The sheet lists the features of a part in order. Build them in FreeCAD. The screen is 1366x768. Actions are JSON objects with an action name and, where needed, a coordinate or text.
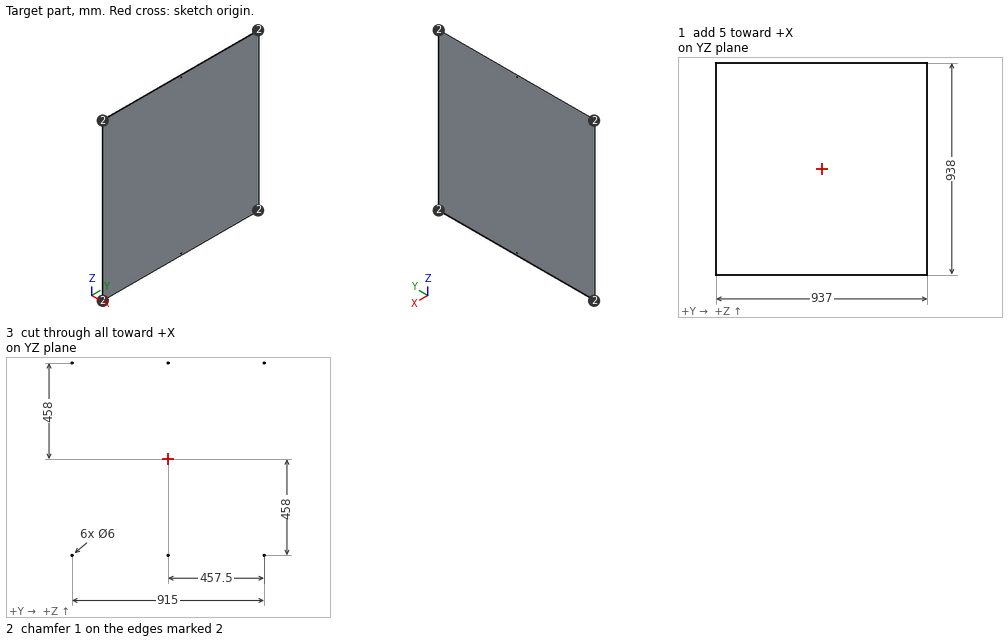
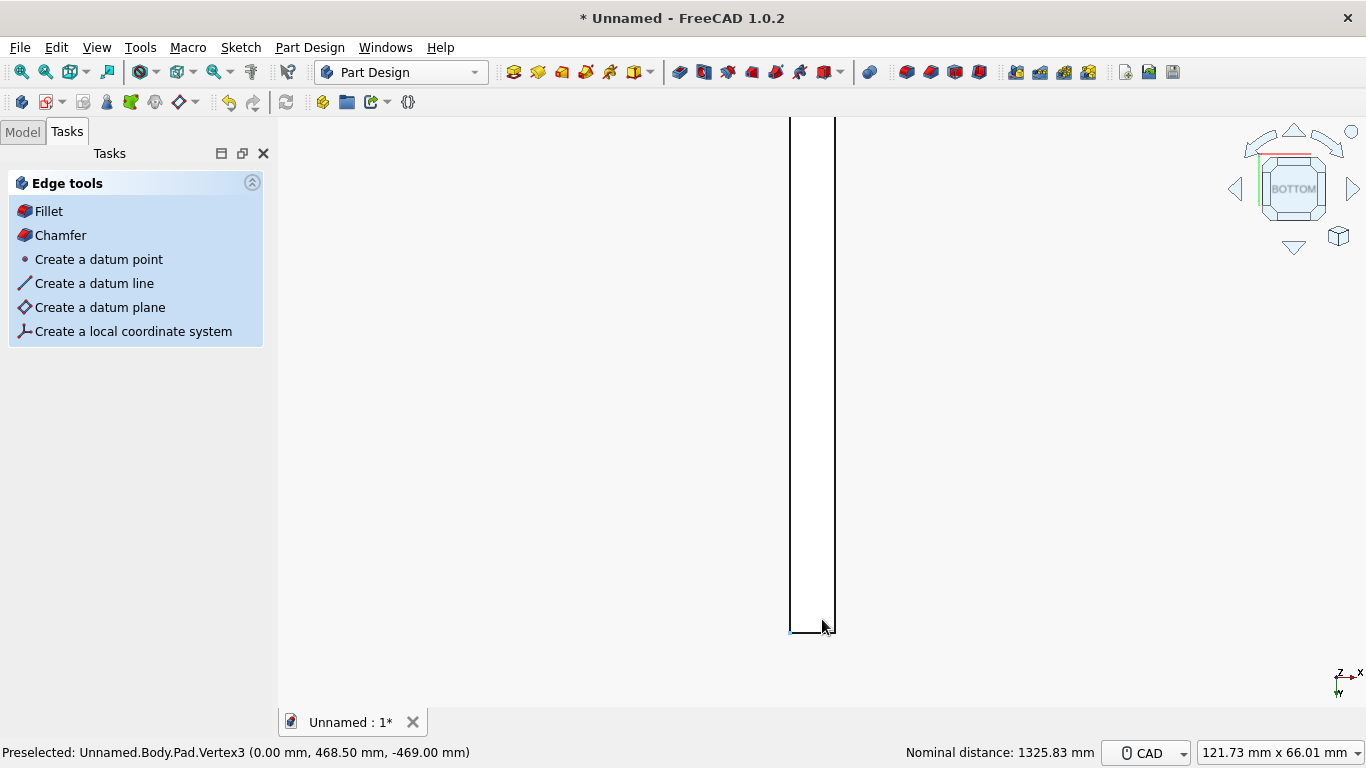
{"action": "left_click", "coordinate": [812, 632], "text": "ctrl"}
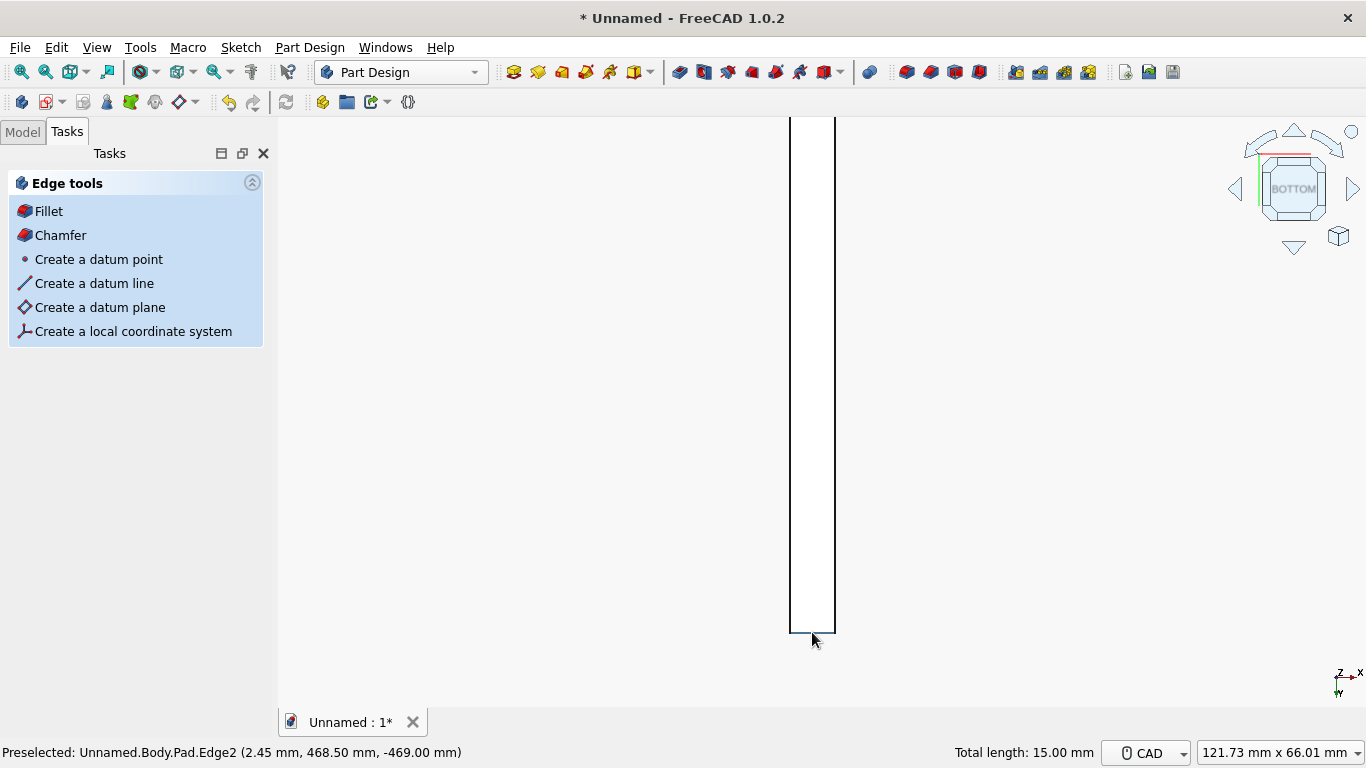
{"action": "left_click", "coordinate": [22, 72]}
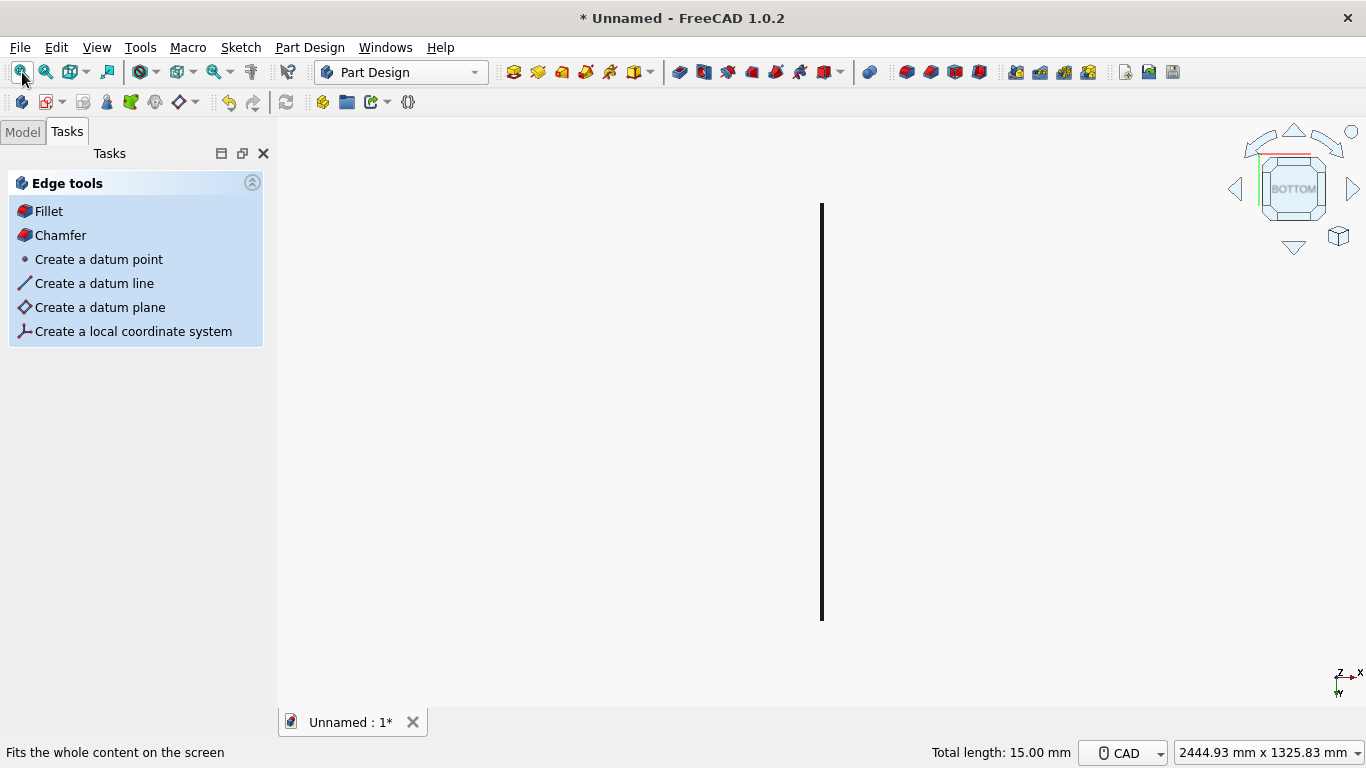
{"action": "key", "text": "4"}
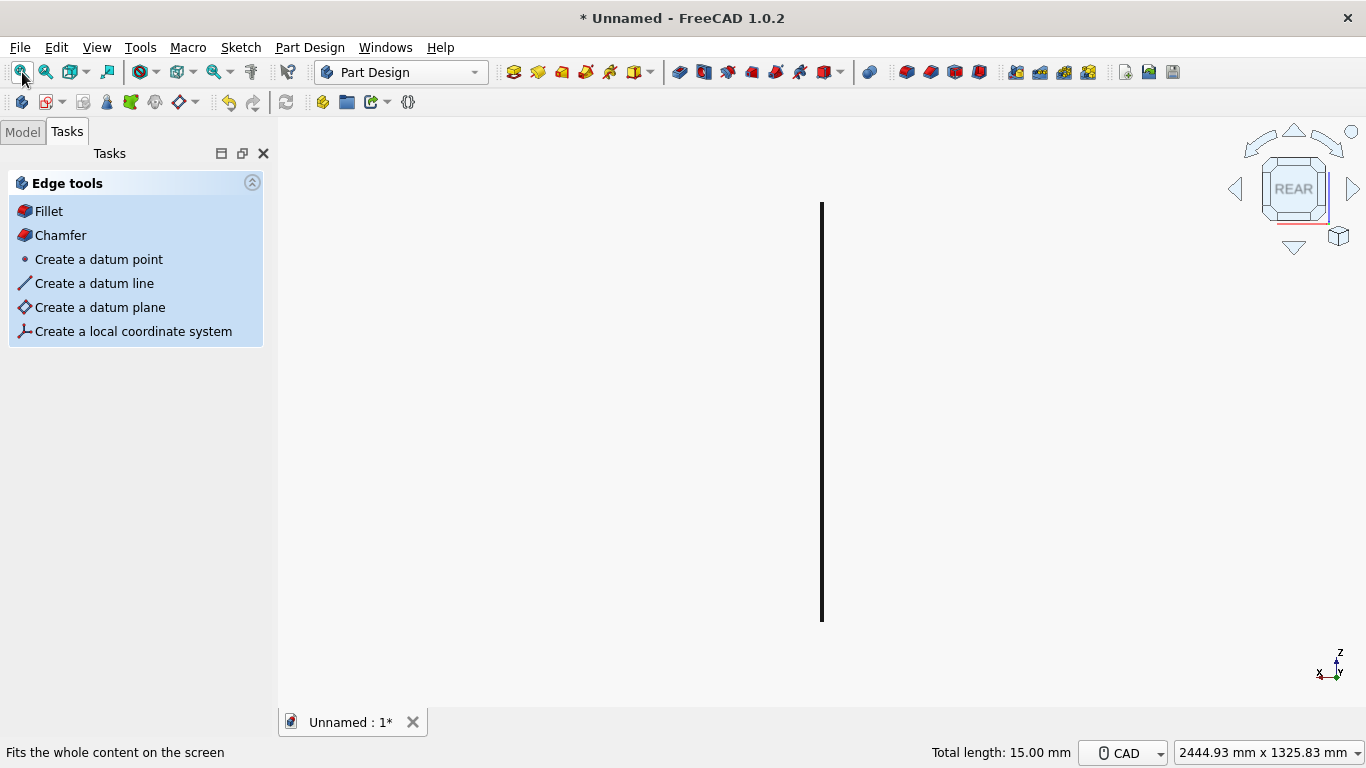
{"action": "scroll", "coordinate": [822, 202], "scroll_direction": "up", "scroll_amount": 15}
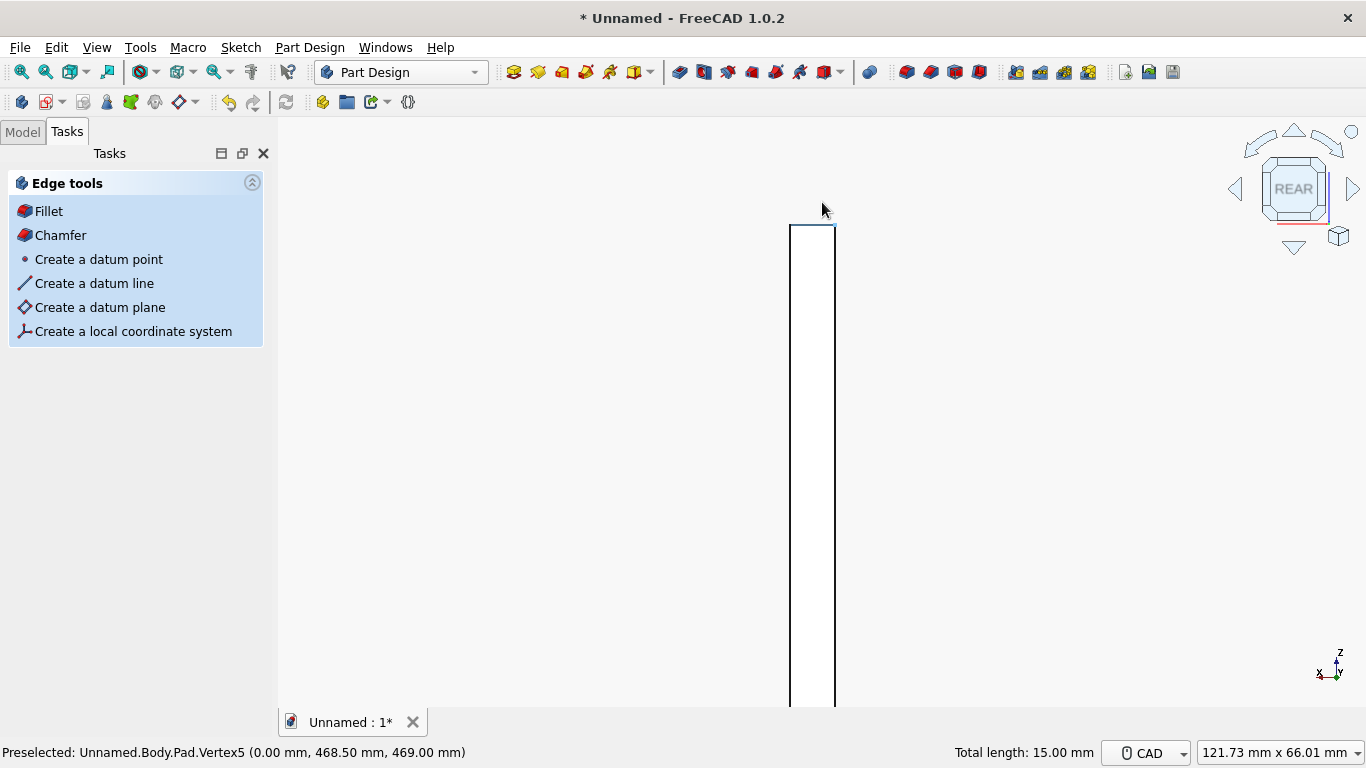
{"action": "left_click", "coordinate": [22, 72]}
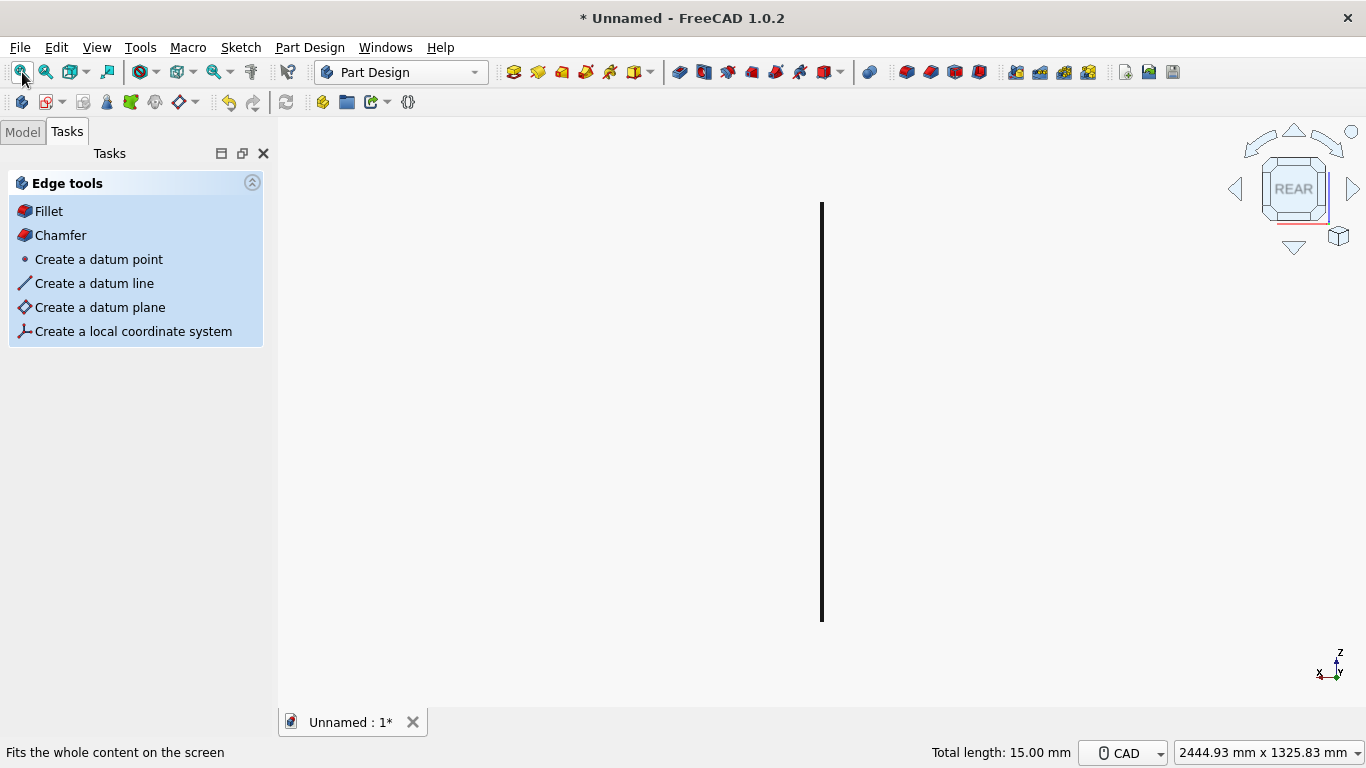
{"action": "key", "text": "6"}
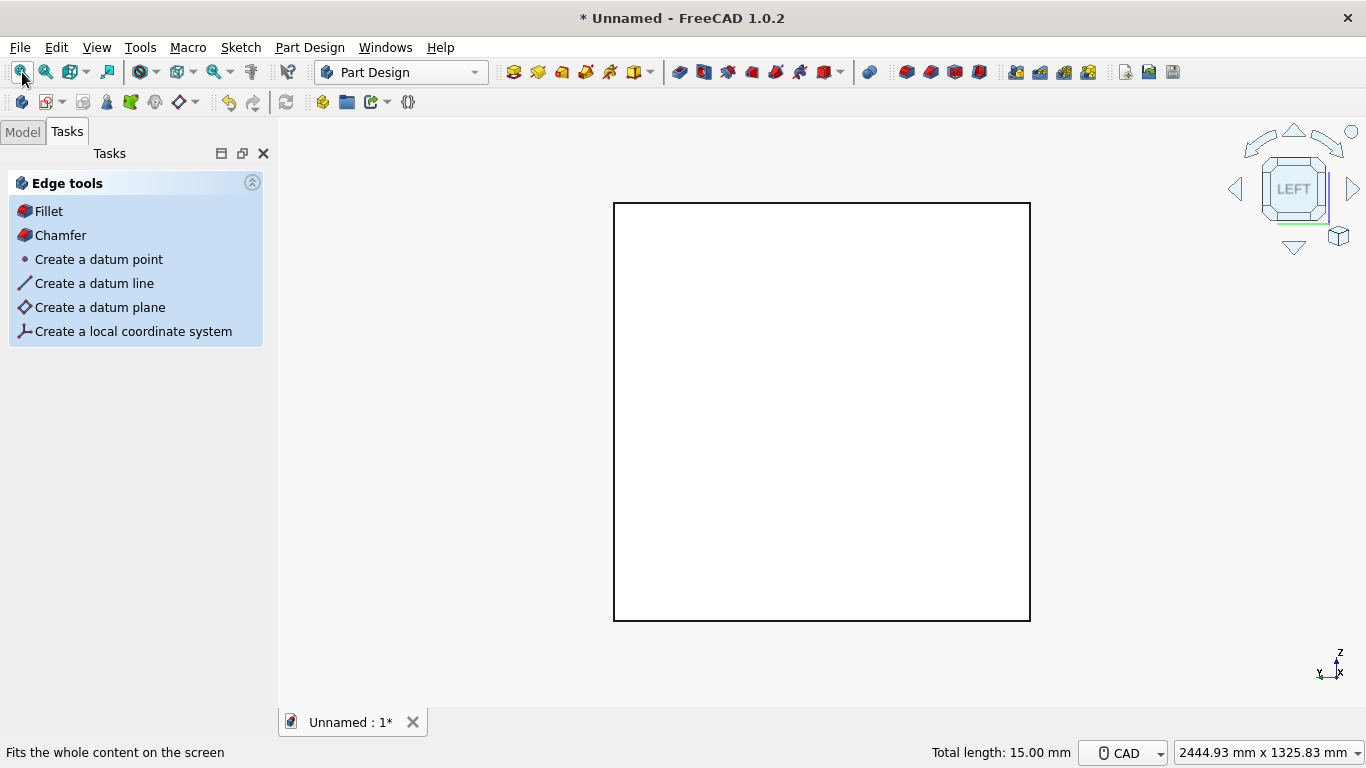
{"action": "scroll", "coordinate": [1030, 202], "scroll_direction": "up", "scroll_amount": 15}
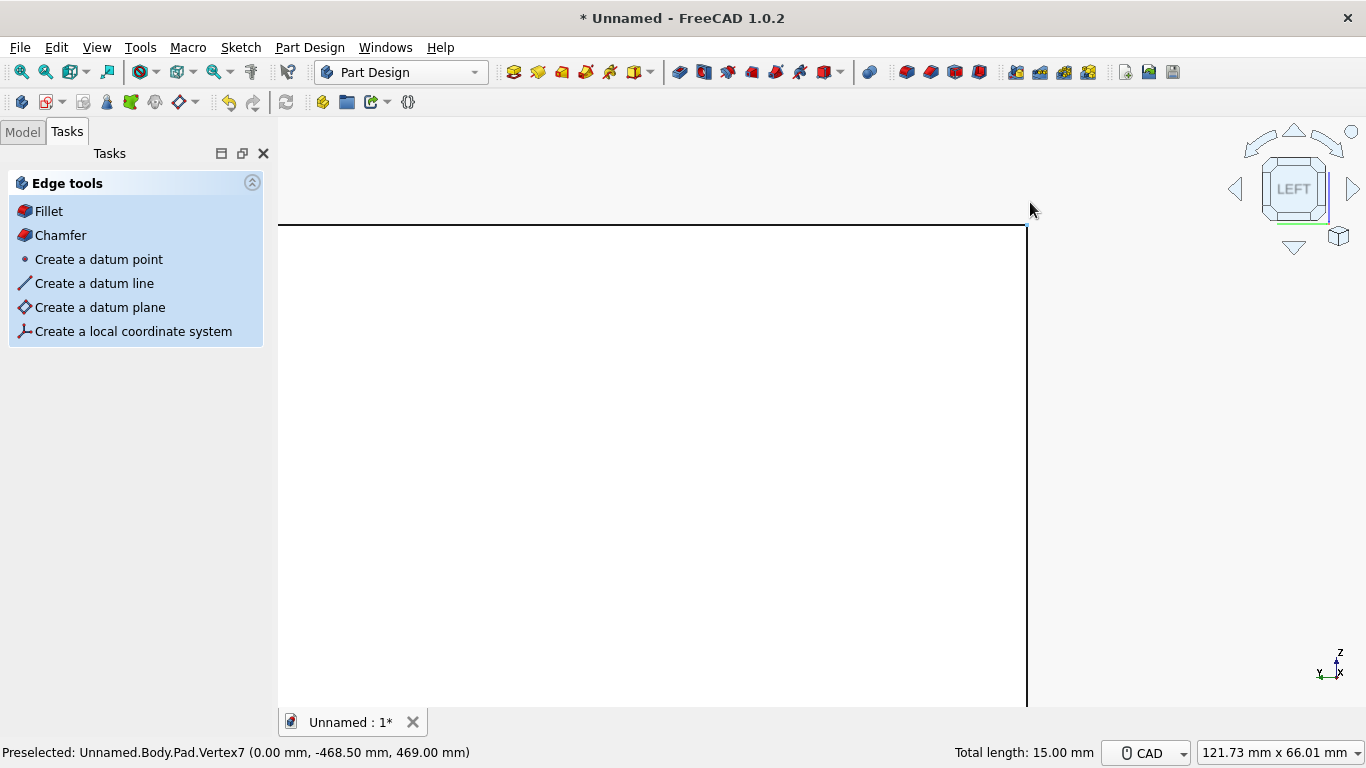
{"action": "left_click", "coordinate": [22, 72]}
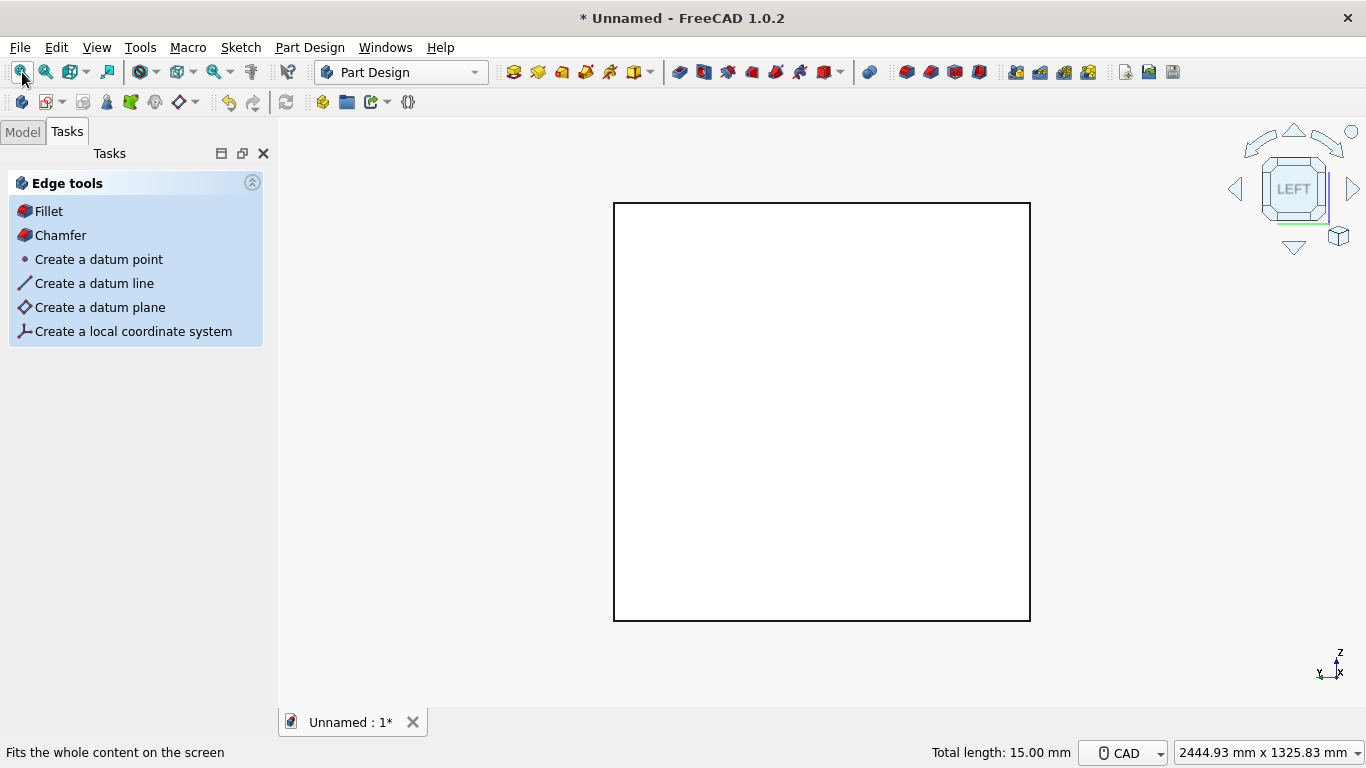
{"action": "key", "text": "v 3"}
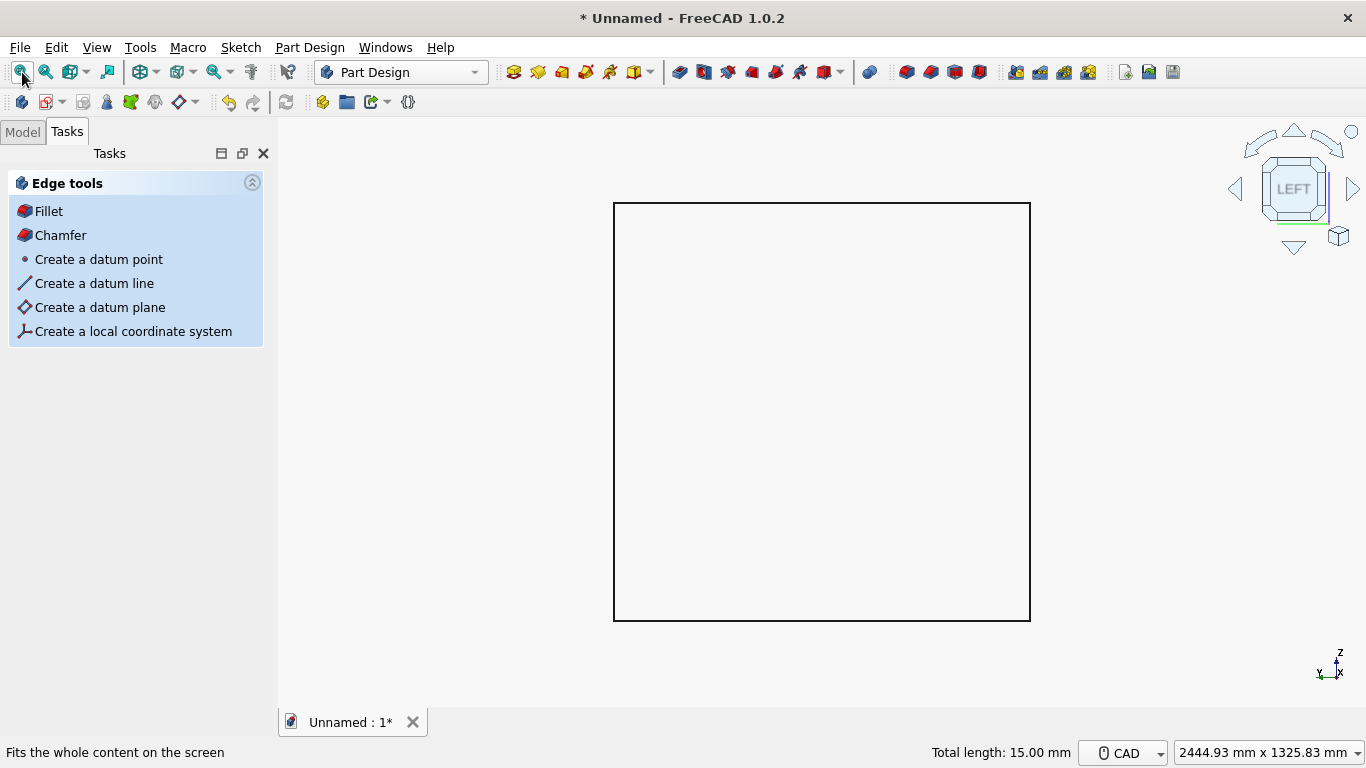
{"action": "key", "text": "0"}